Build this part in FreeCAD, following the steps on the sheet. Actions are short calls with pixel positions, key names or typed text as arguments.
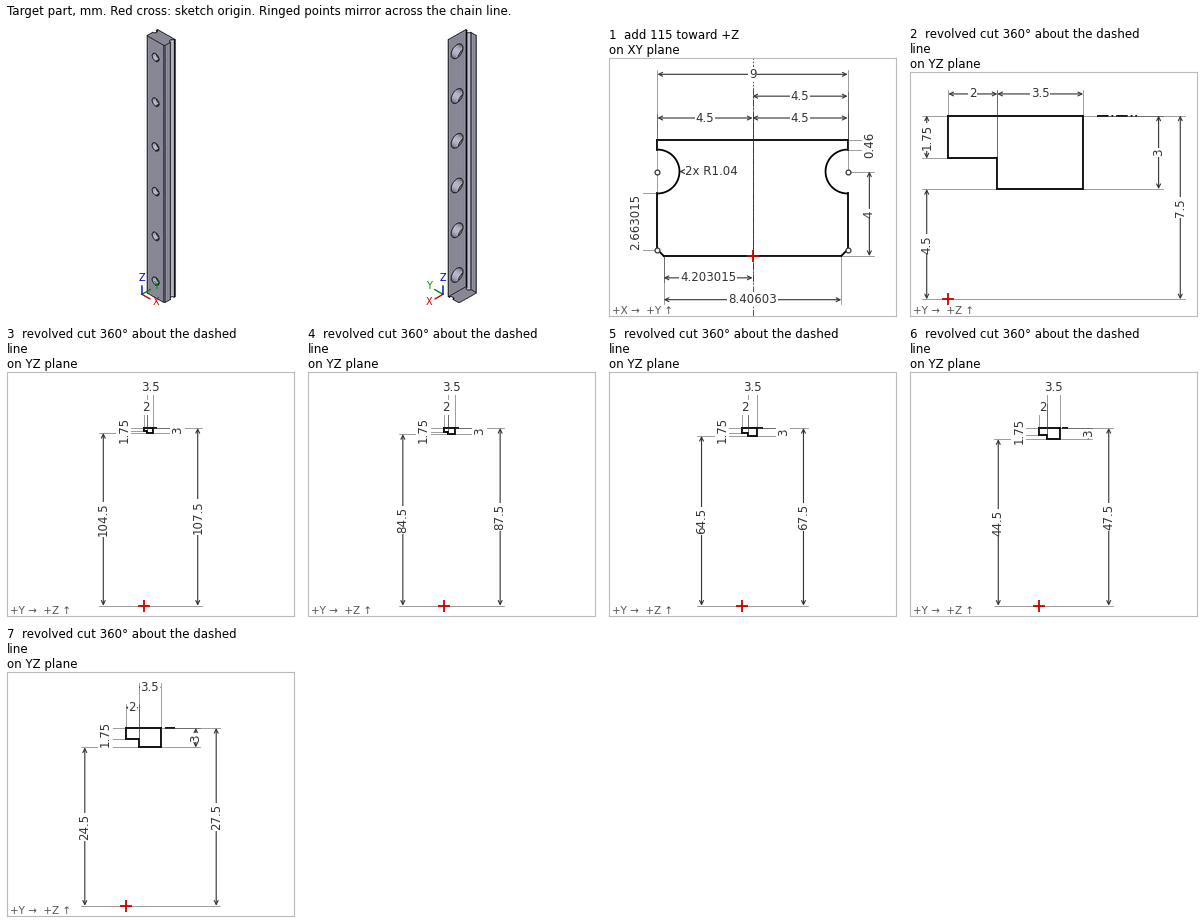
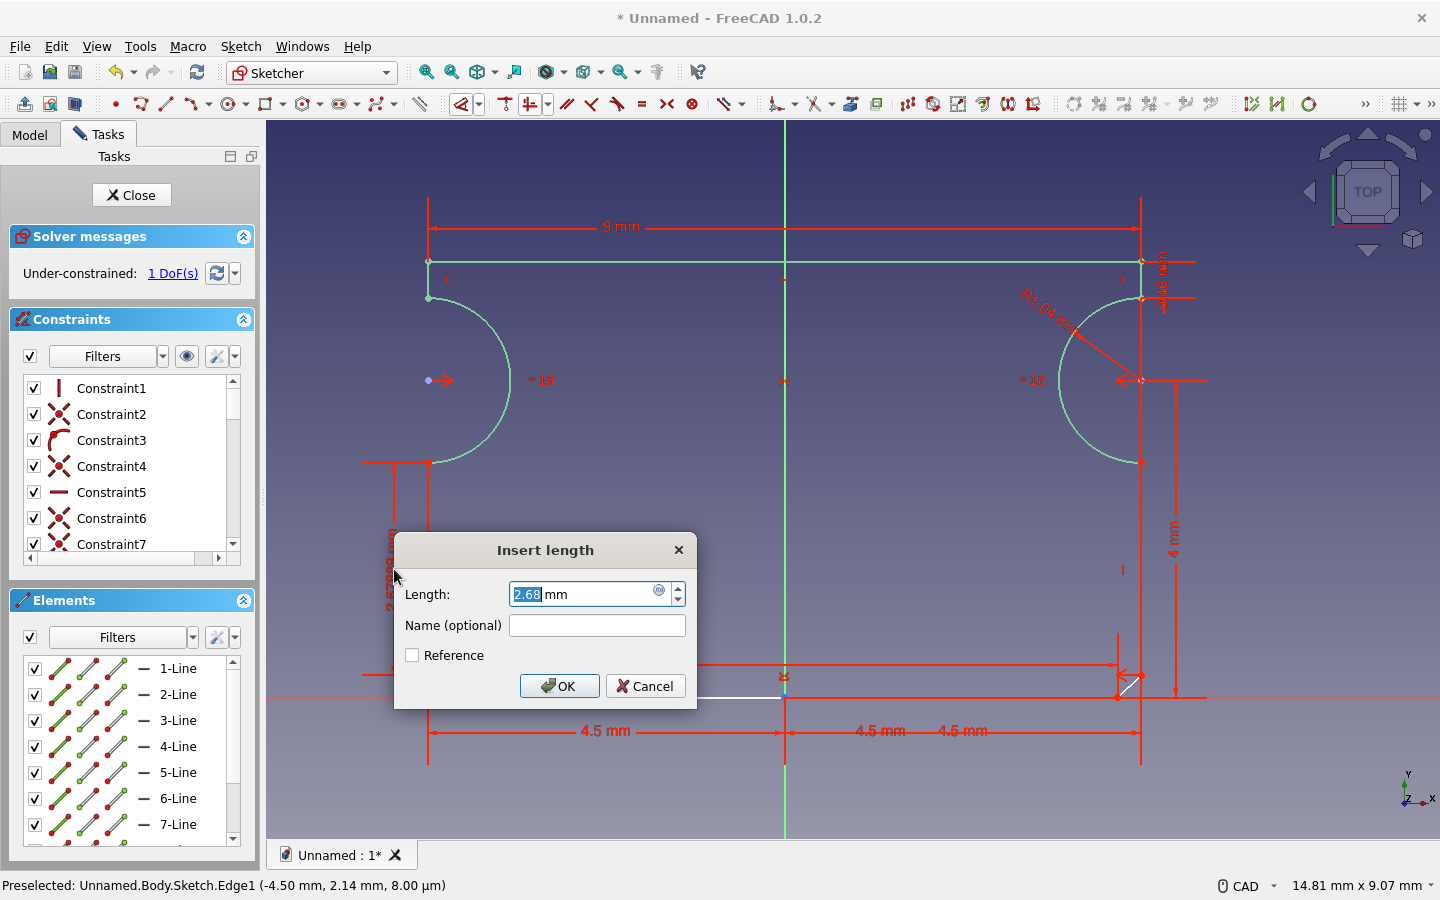
text(2.663015)
key(Return)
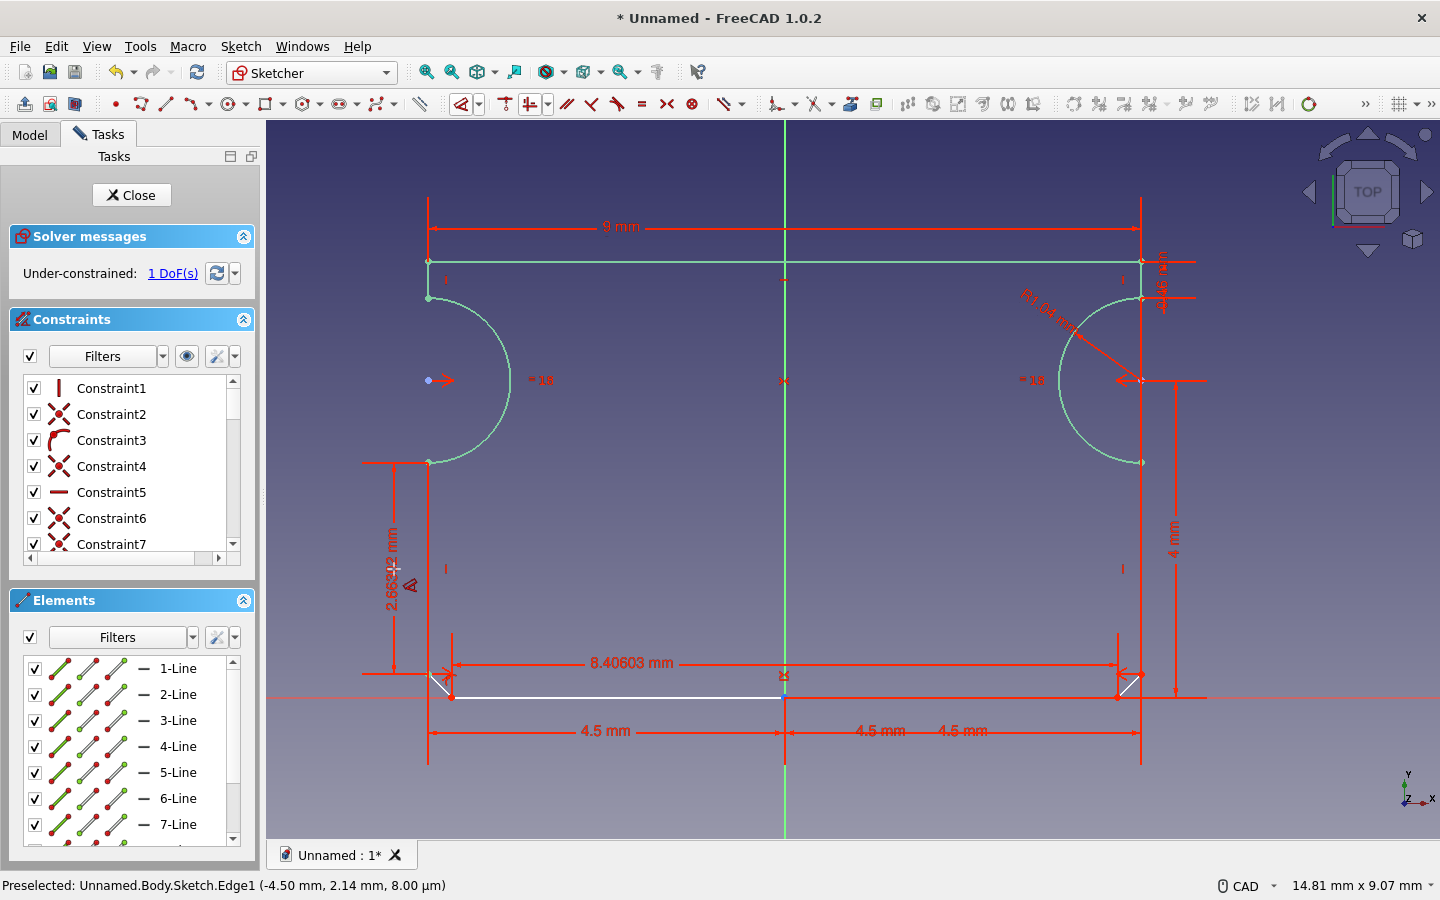
click(452, 698)
click(695, 732)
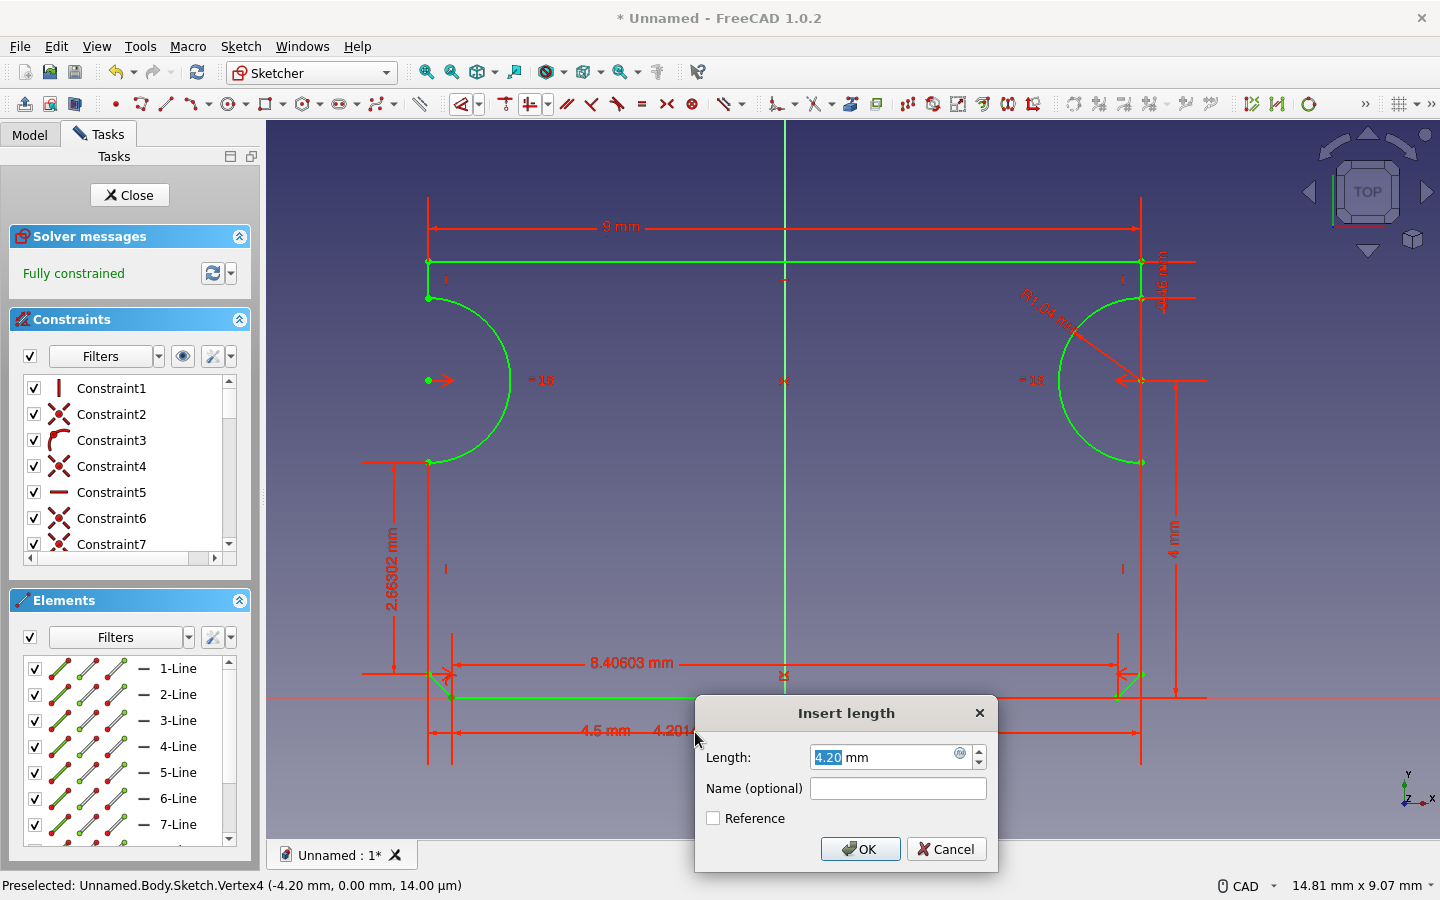
text(4.203015)
key(Return)
key(Escape)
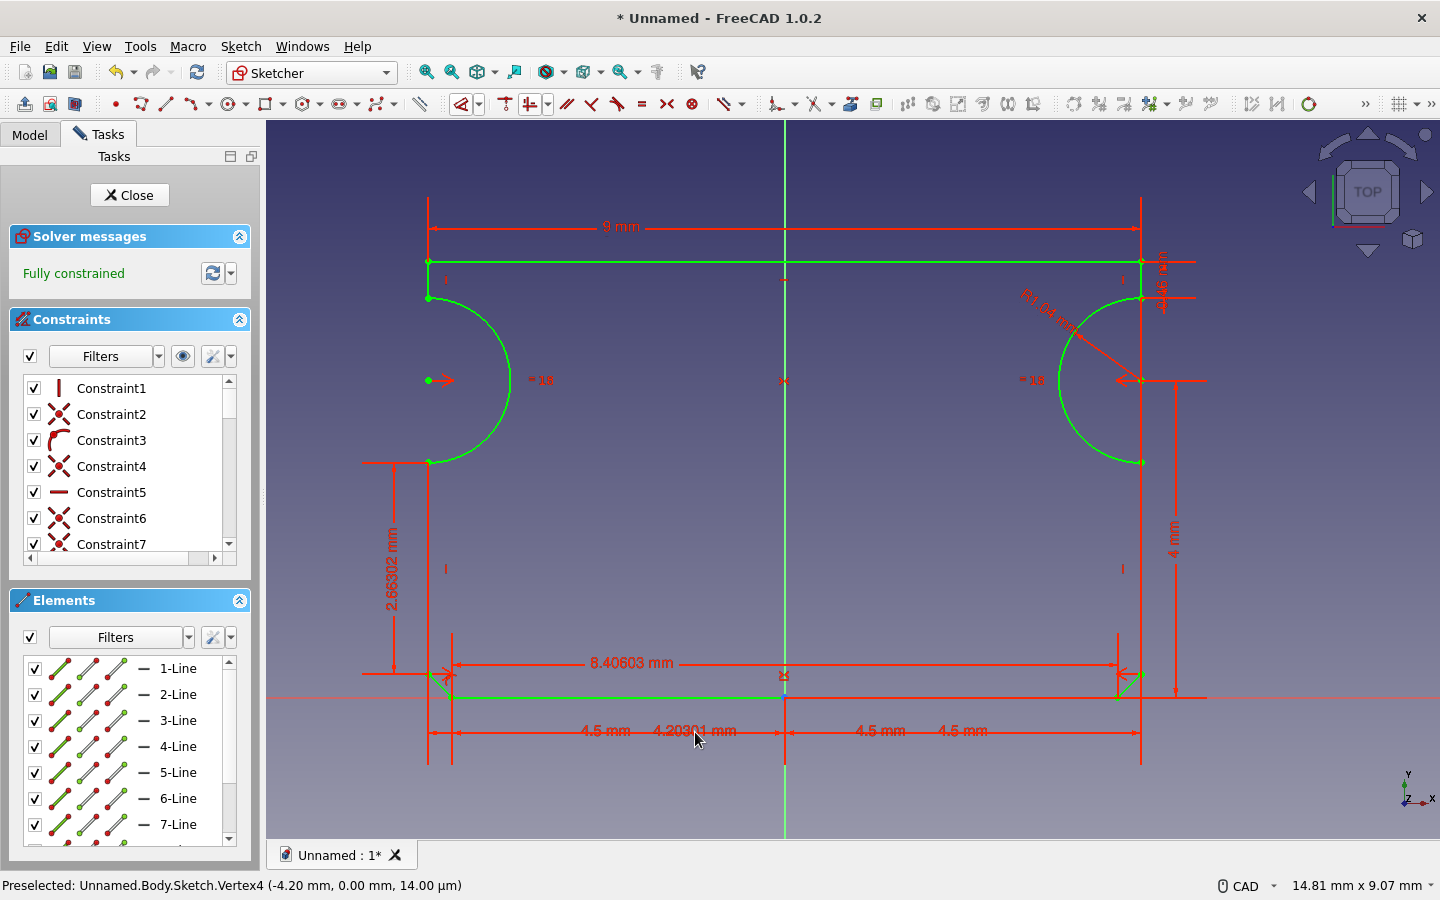
click(130, 195)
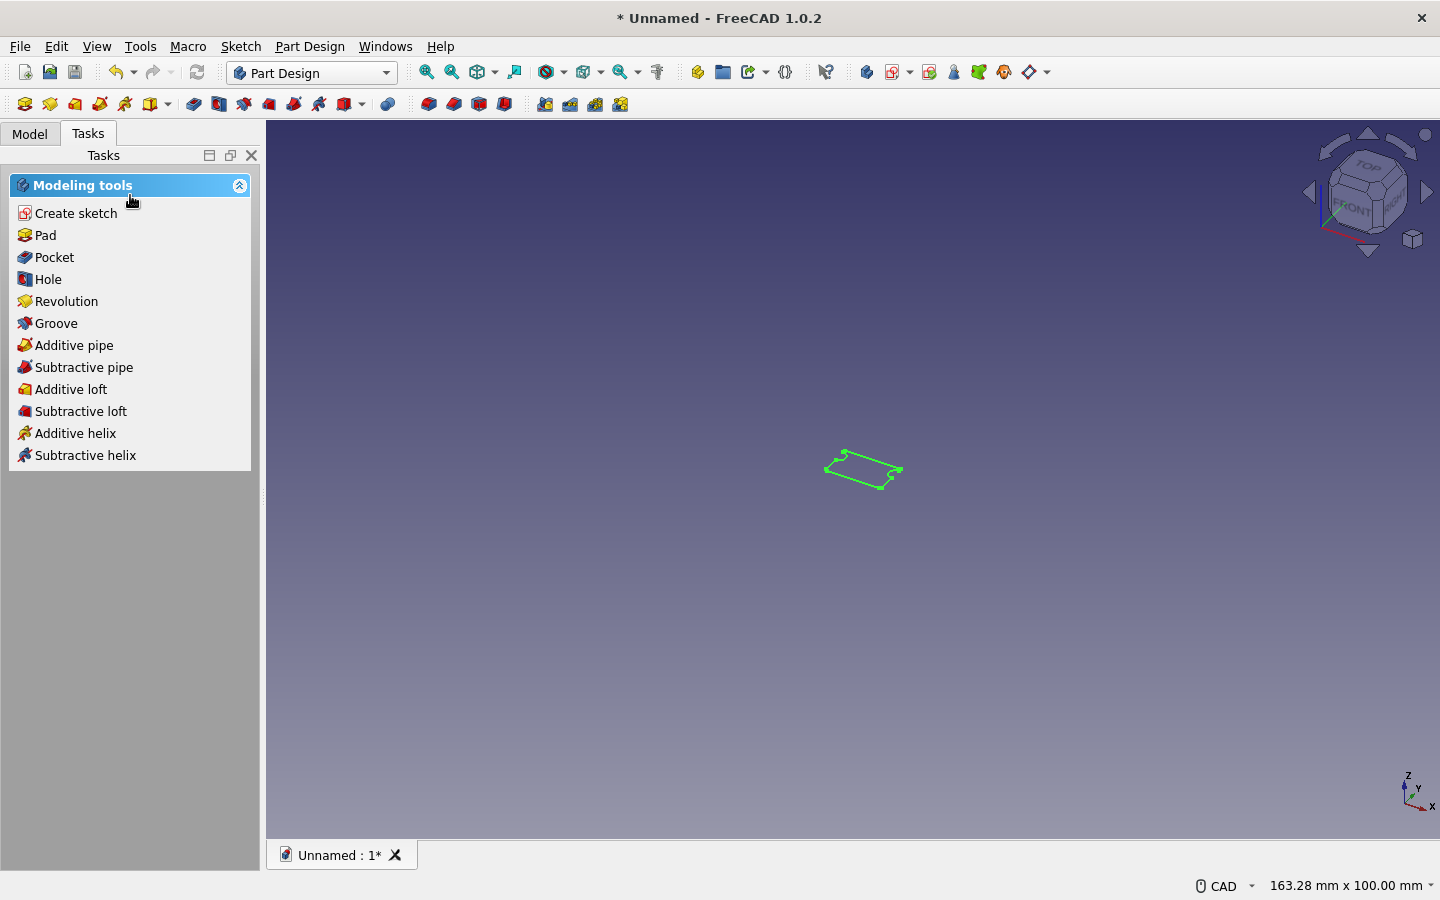
click(25, 104)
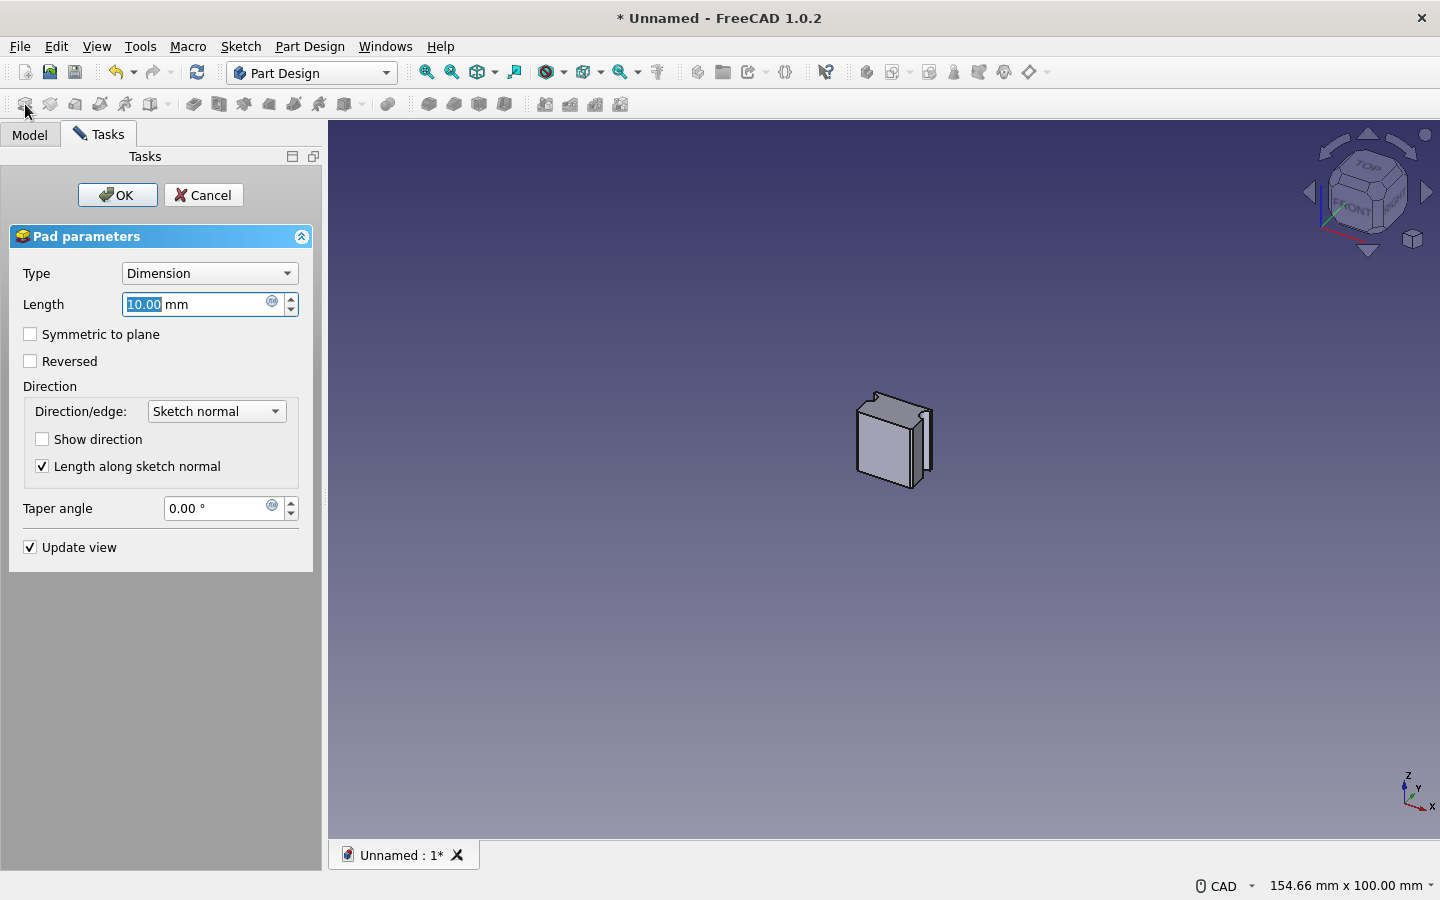
text(115)
key(Tab)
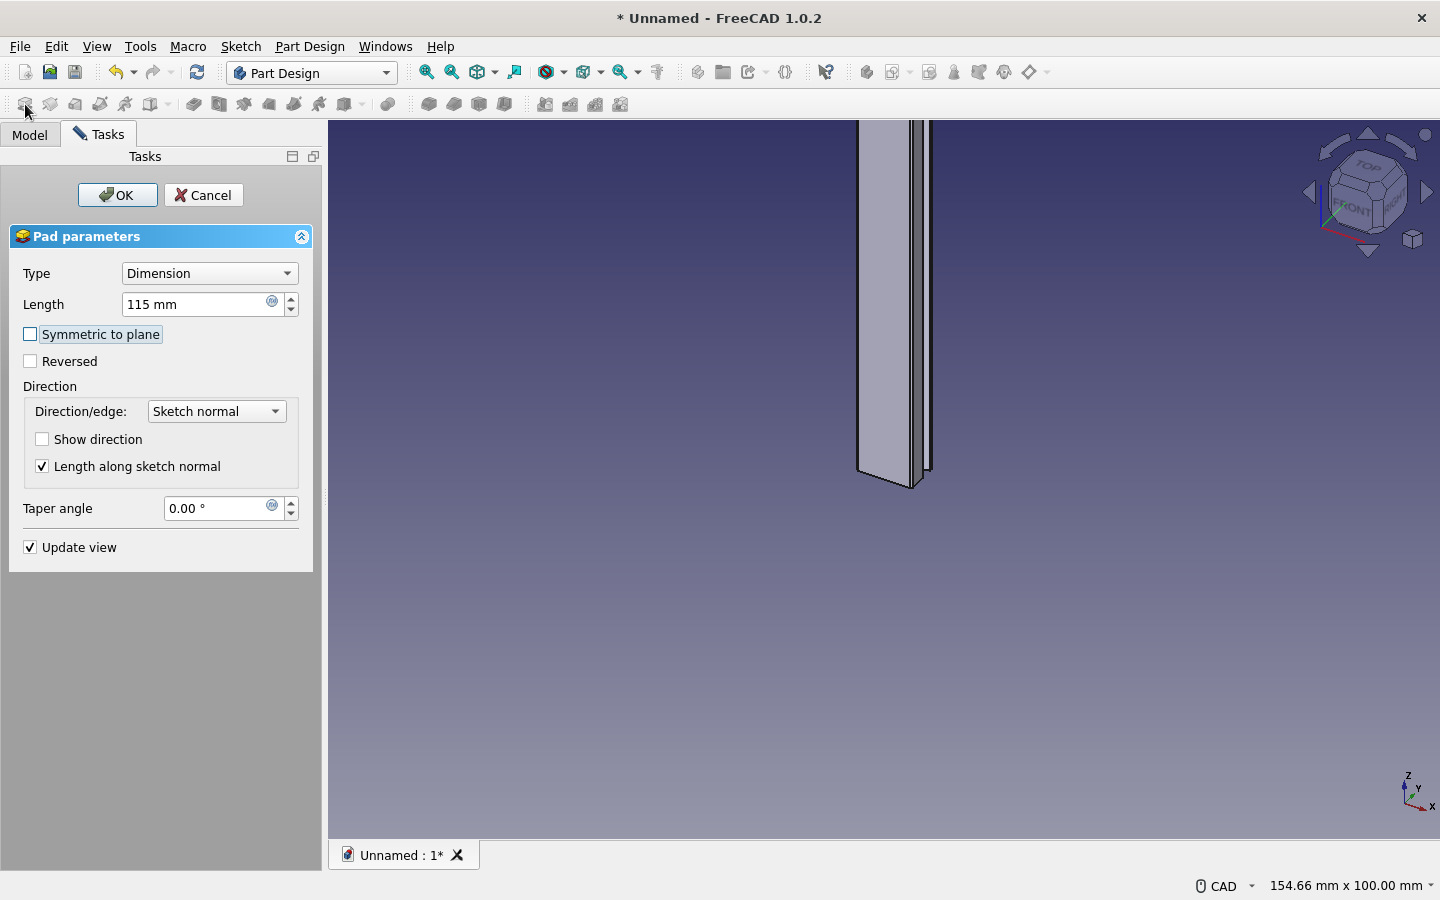
click(118, 195)